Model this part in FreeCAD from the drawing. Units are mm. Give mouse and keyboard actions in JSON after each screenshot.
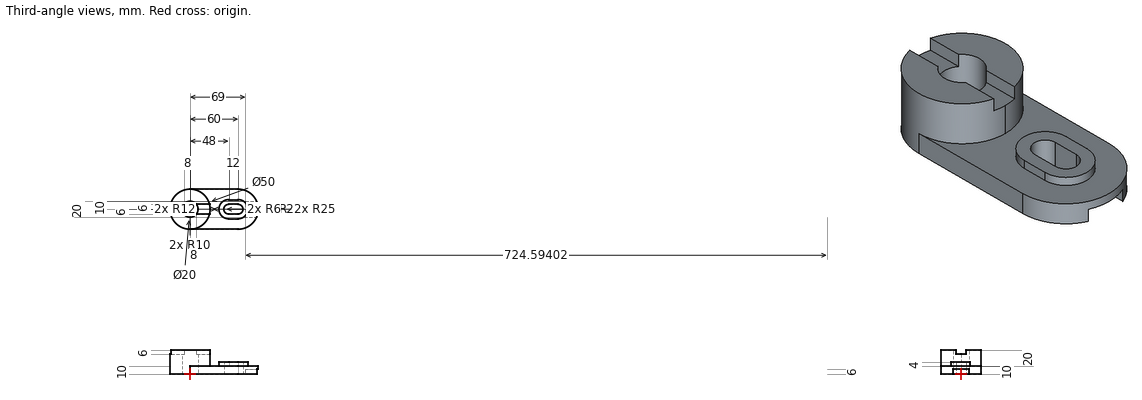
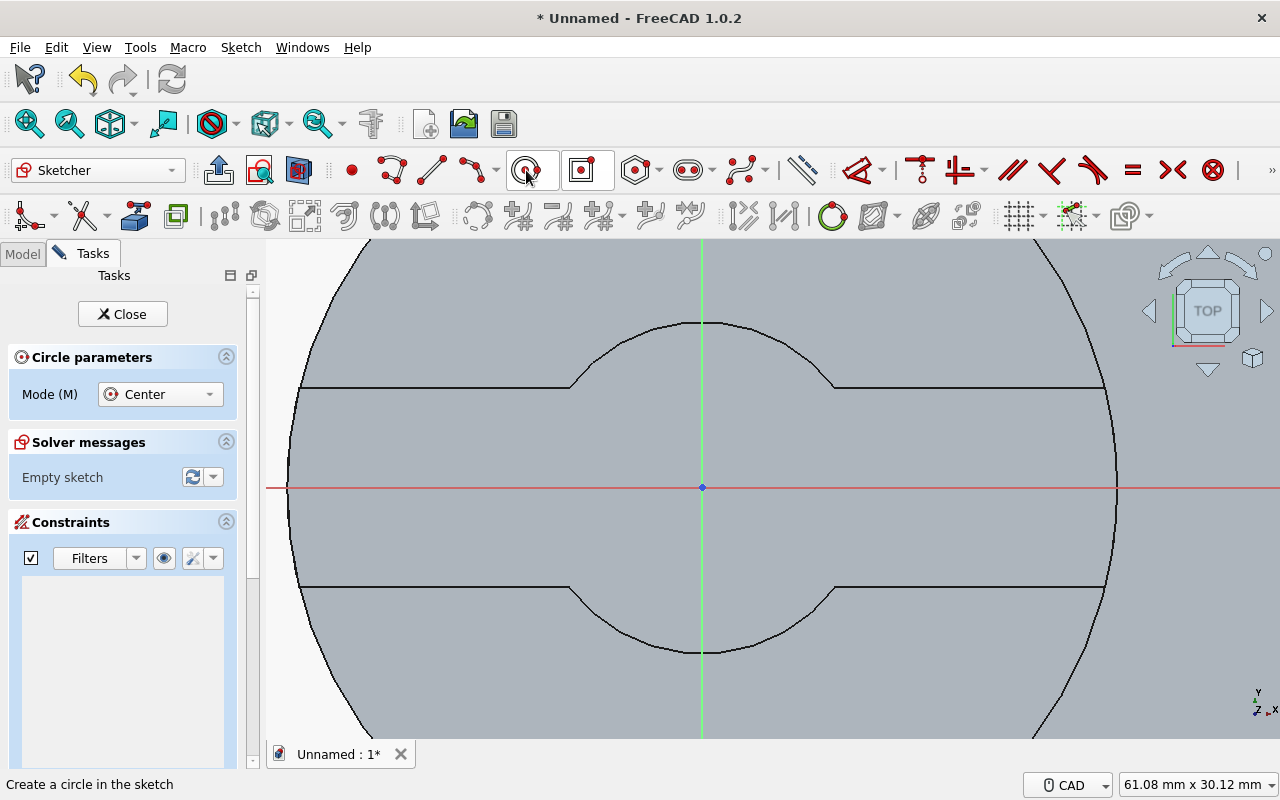
{"action": "left_click", "coordinate": [702, 488]}
{"action": "left_click", "coordinate": [820, 370]}
{"action": "key", "text": "Escape"}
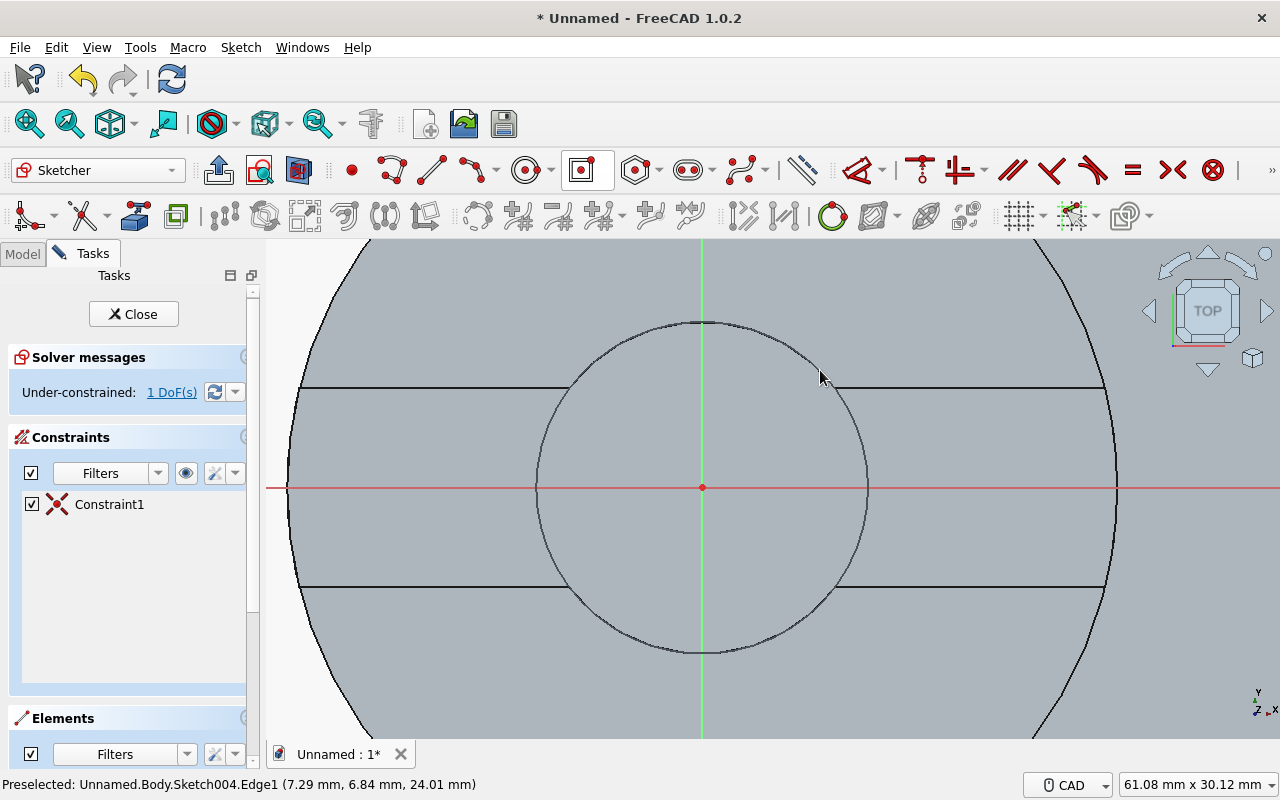
{"action": "left_click", "coordinate": [858, 170]}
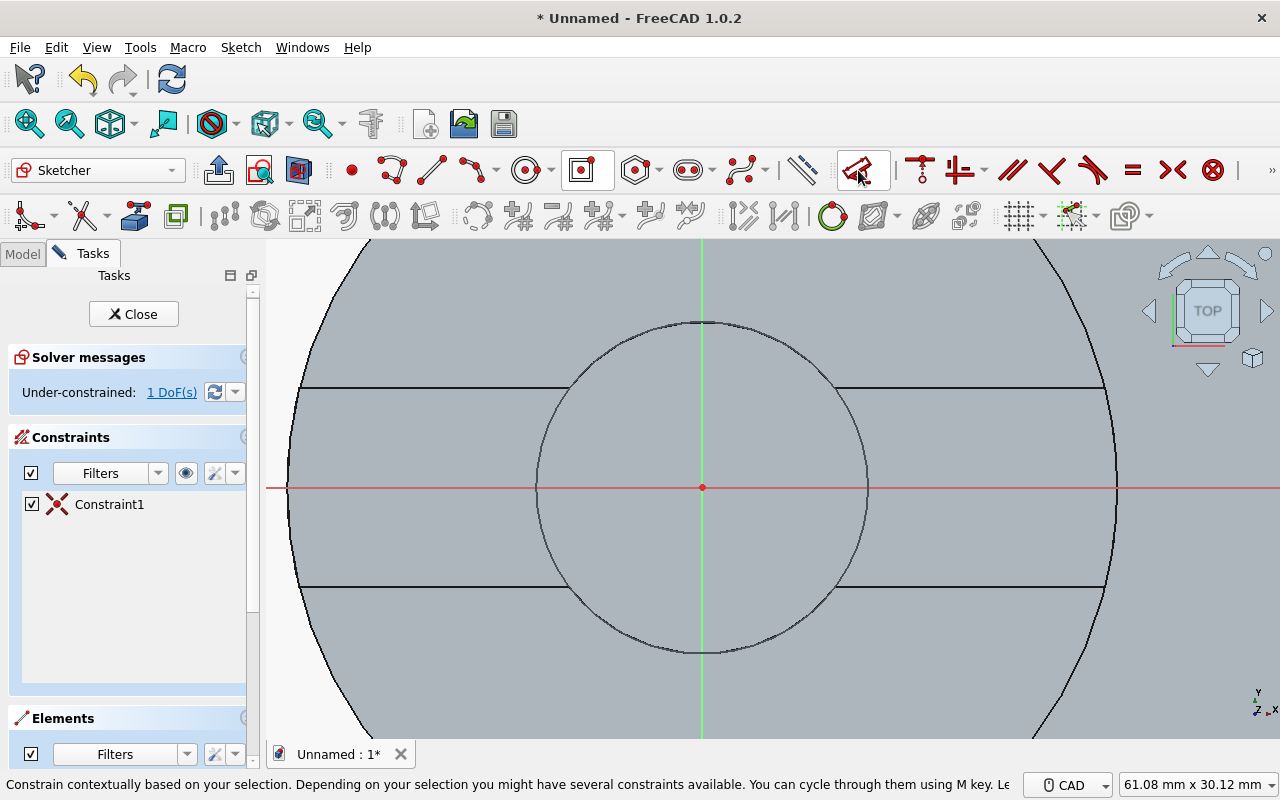
{"action": "left_click", "coordinate": [819, 370]}
{"action": "left_click", "coordinate": [842, 347]}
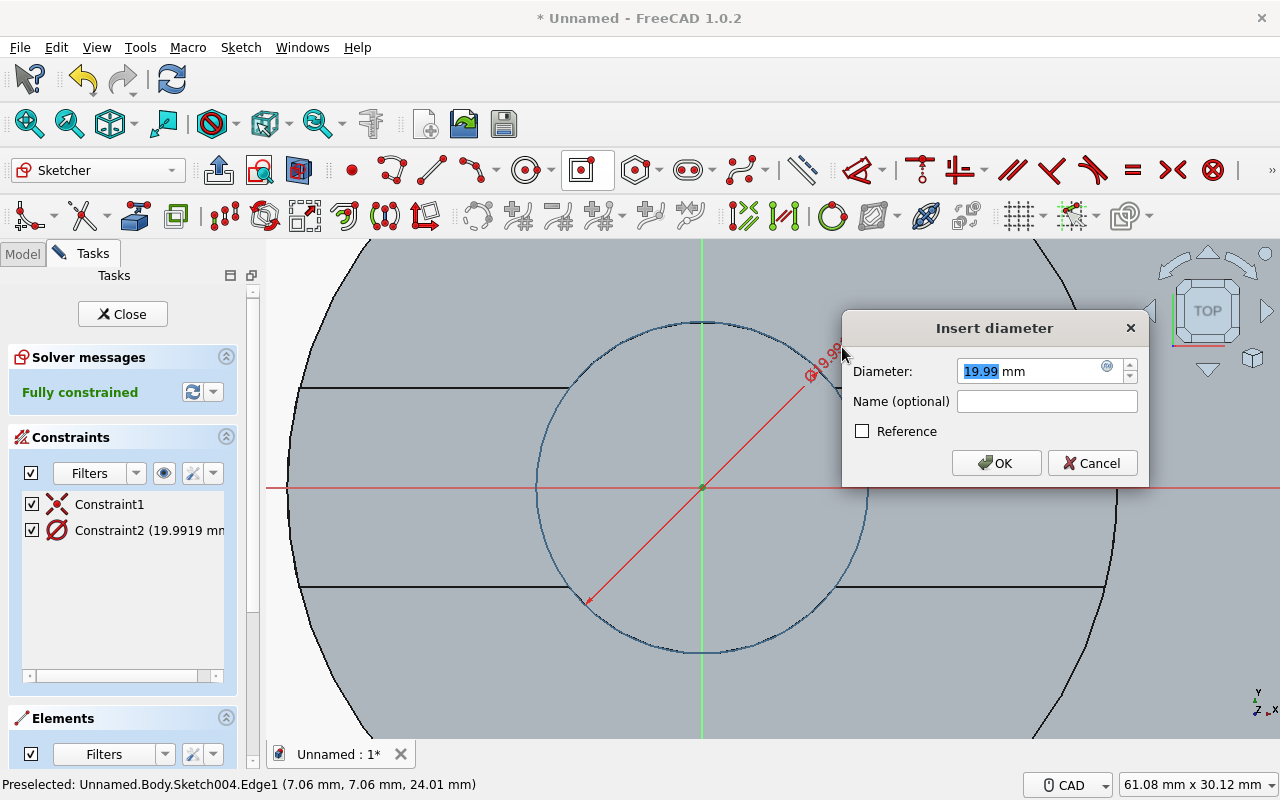
{"action": "type", "text": "20"}
{"action": "key", "text": "Return"}
{"action": "key", "text": "Escape"}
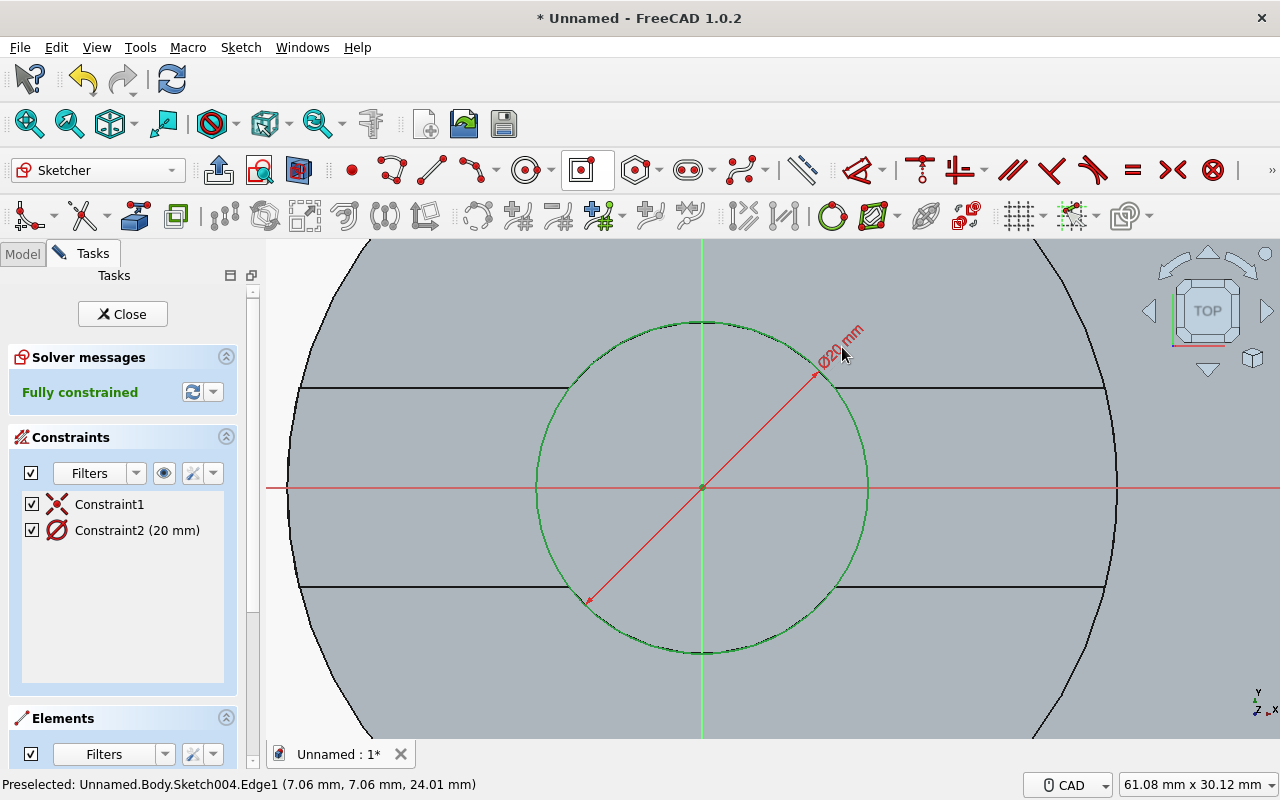
{"action": "left_click", "coordinate": [123, 314]}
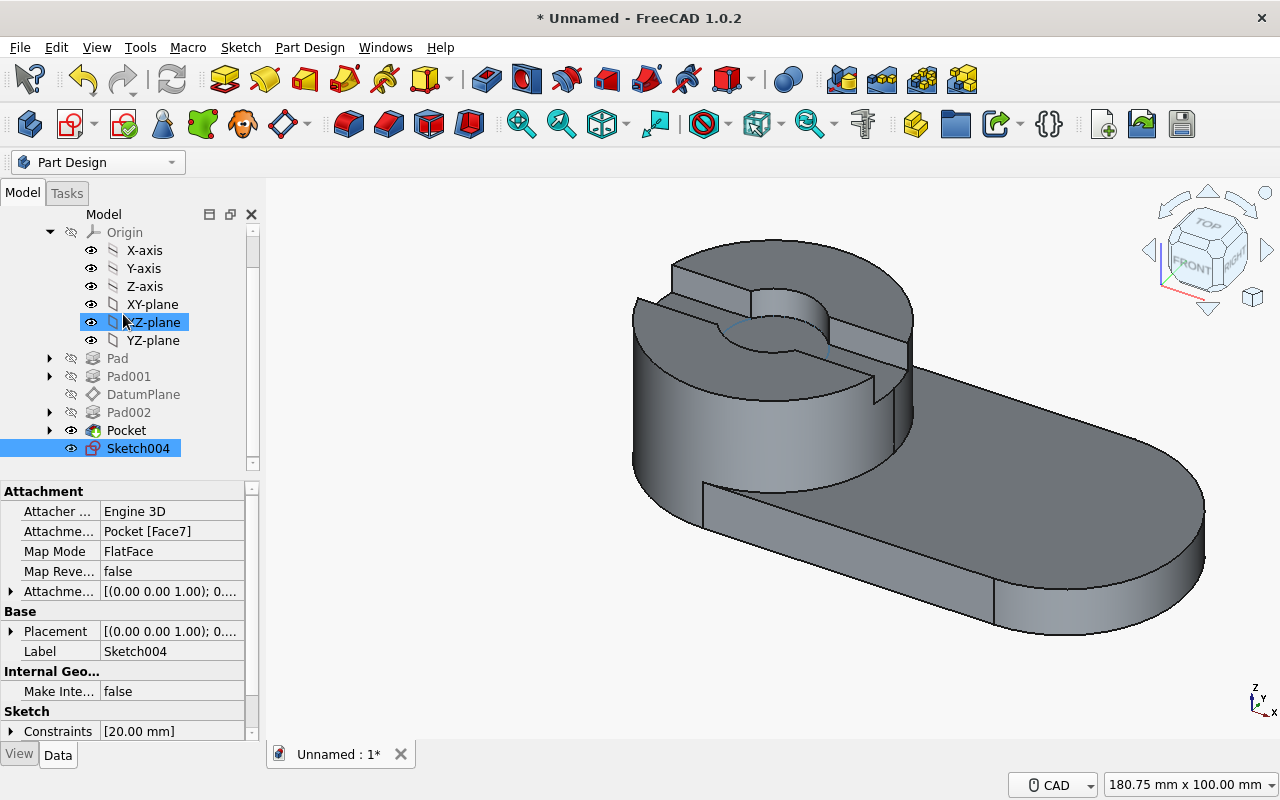
{"action": "left_click", "coordinate": [488, 80]}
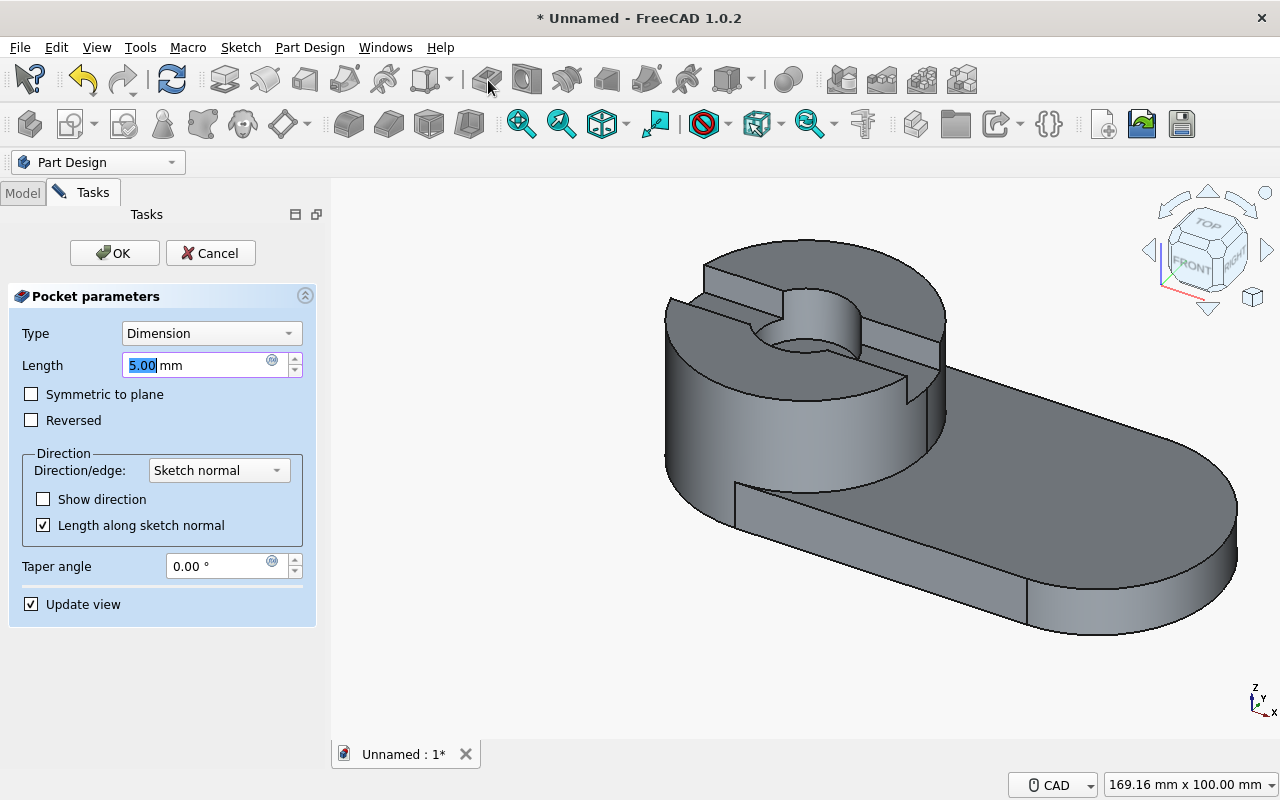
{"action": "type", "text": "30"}
{"action": "key", "text": "Tab"}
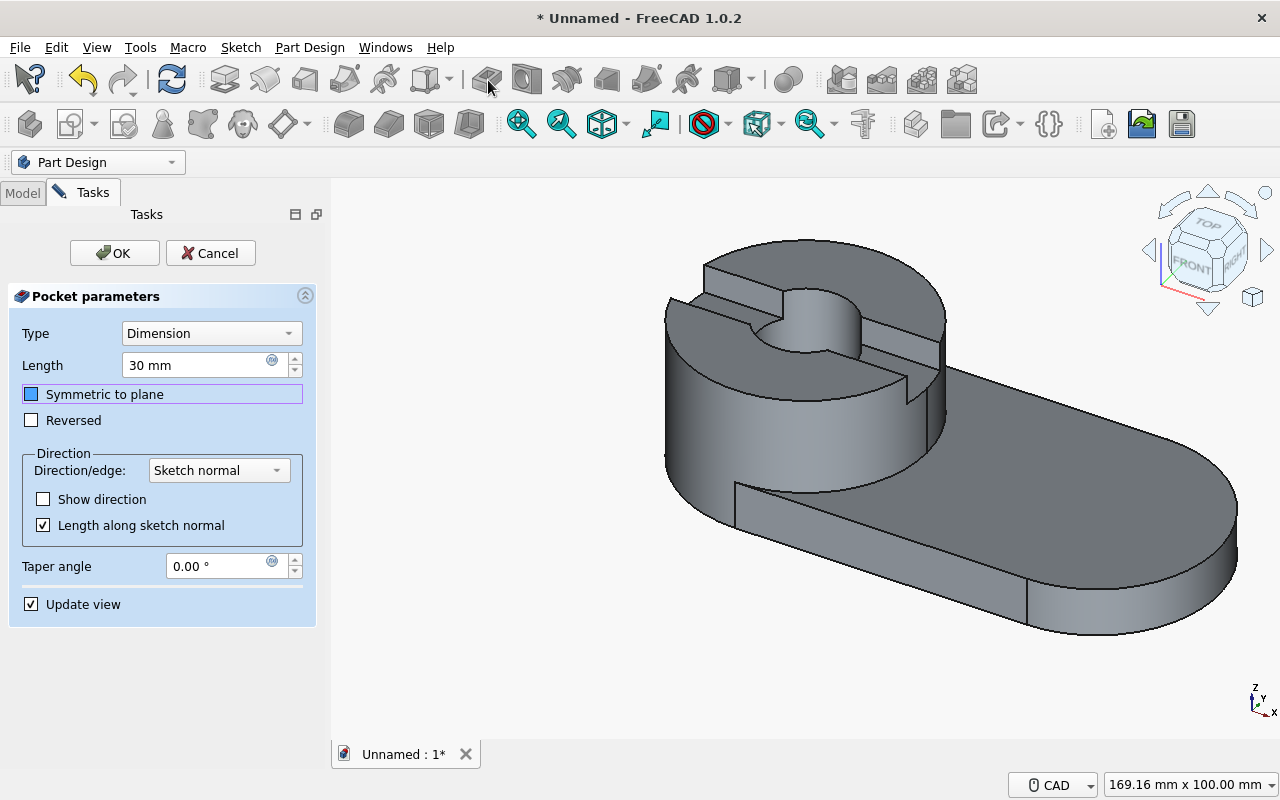
{"action": "left_click", "coordinate": [115, 253]}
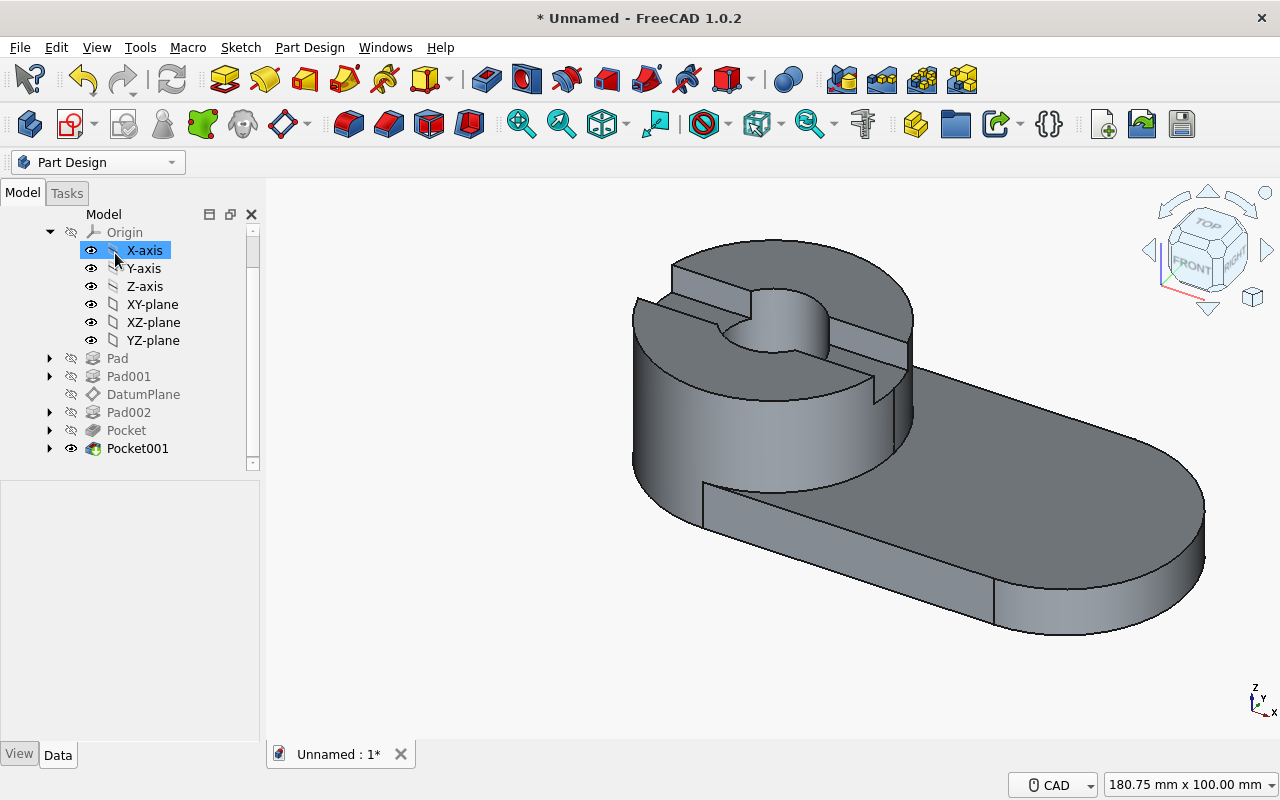
{"action": "left_click", "coordinate": [1038, 499]}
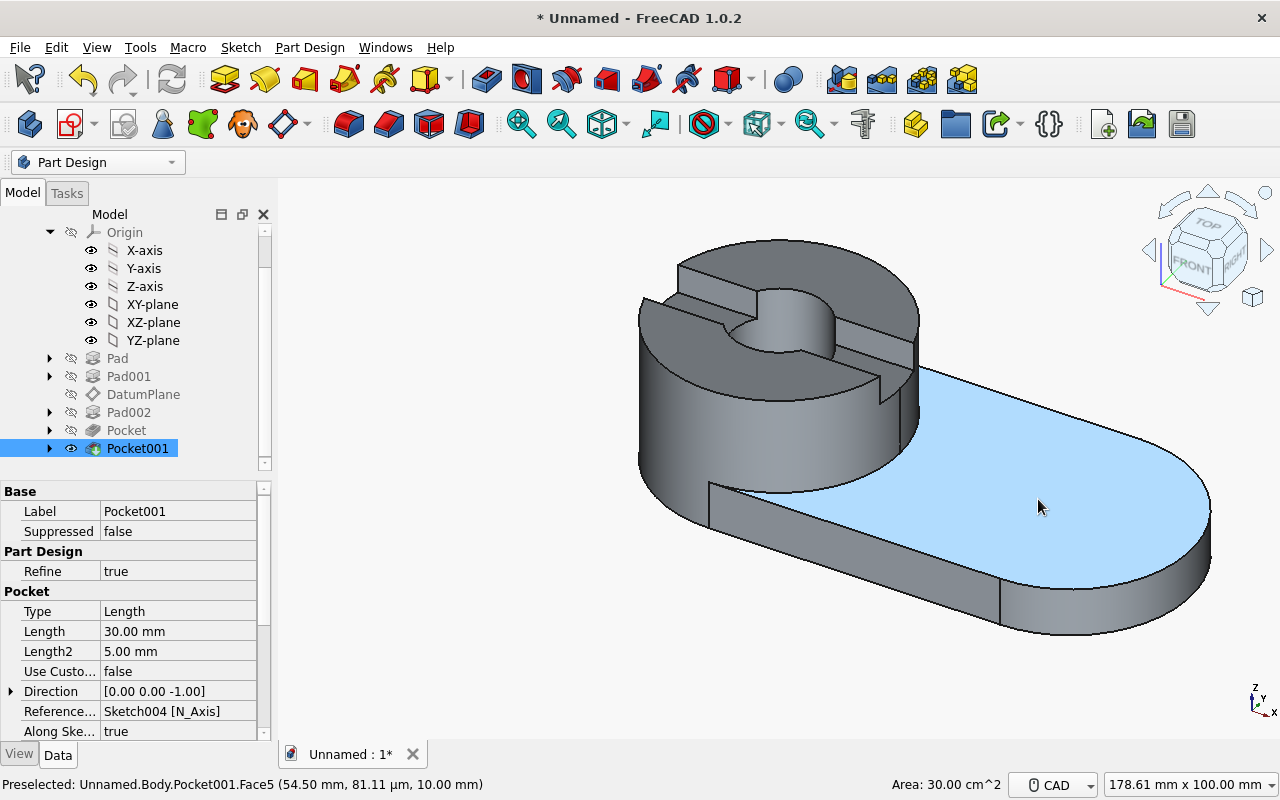
{"action": "left_click", "coordinate": [70, 124]}